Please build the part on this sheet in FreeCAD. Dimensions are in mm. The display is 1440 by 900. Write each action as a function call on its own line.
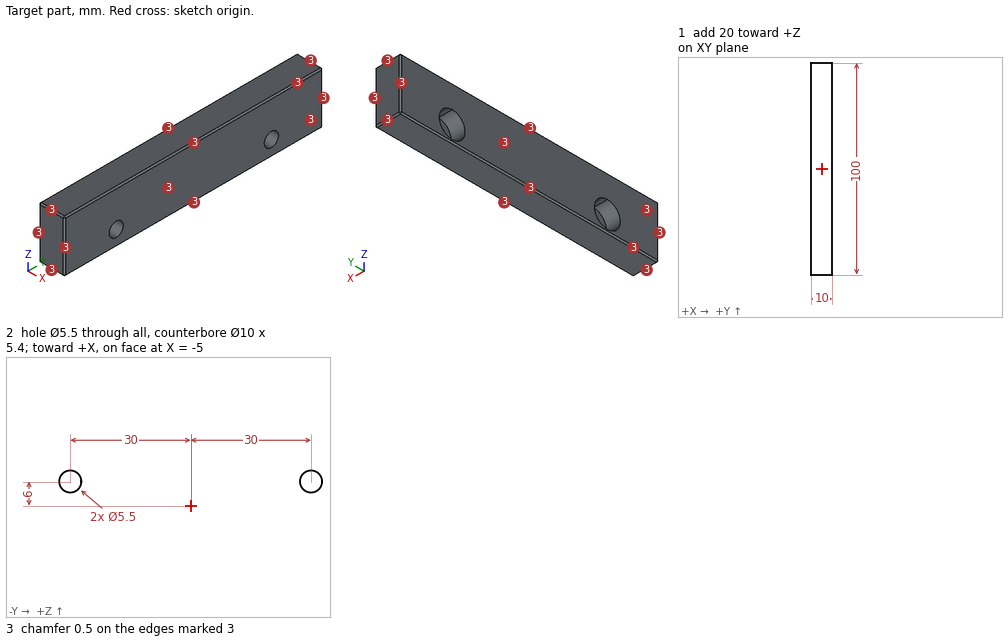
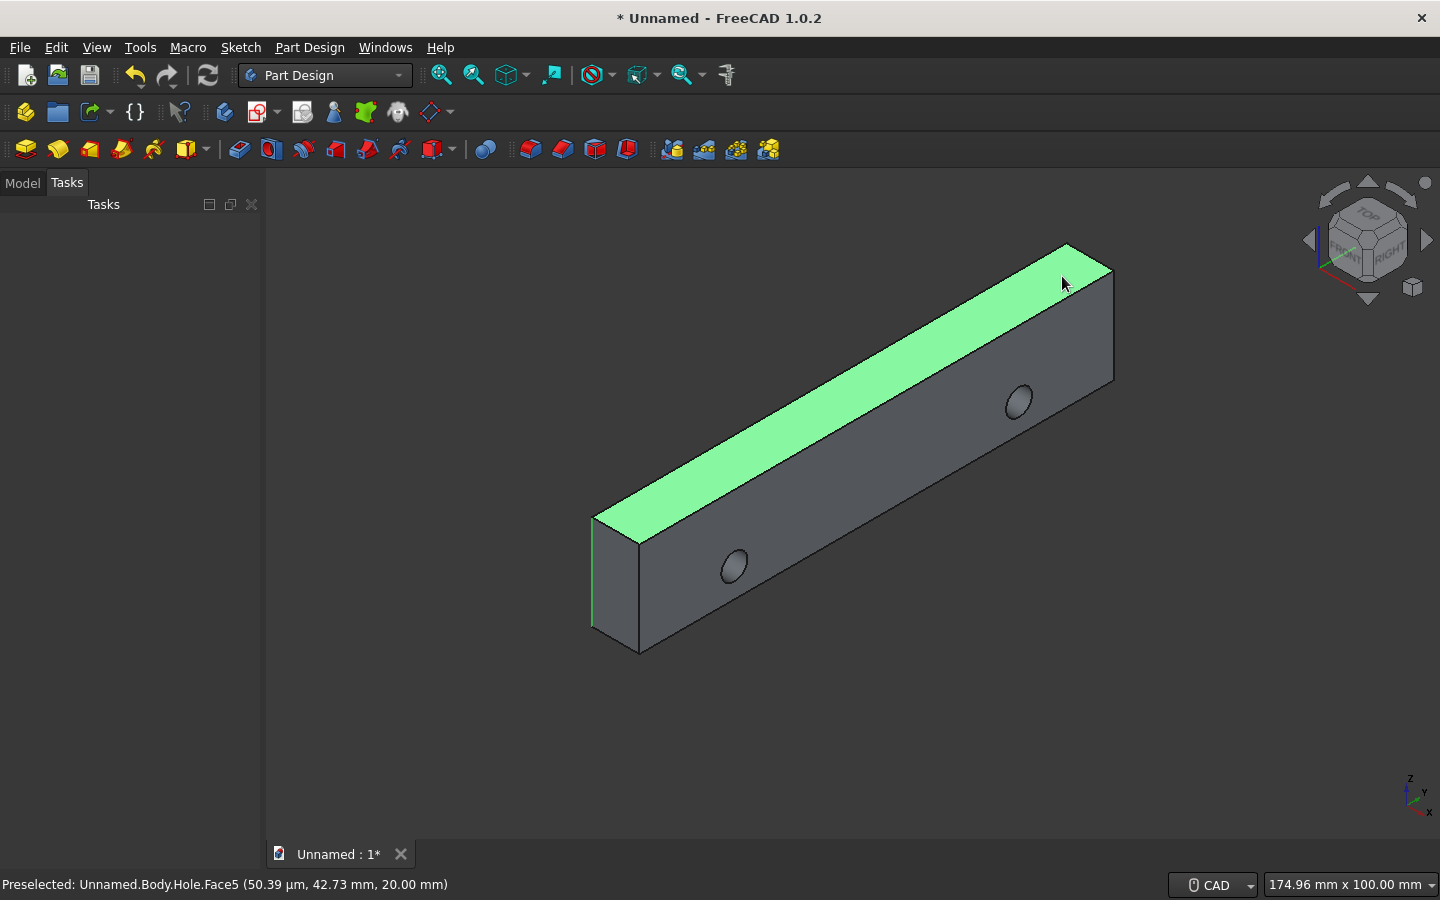
click(639, 598, ctrl)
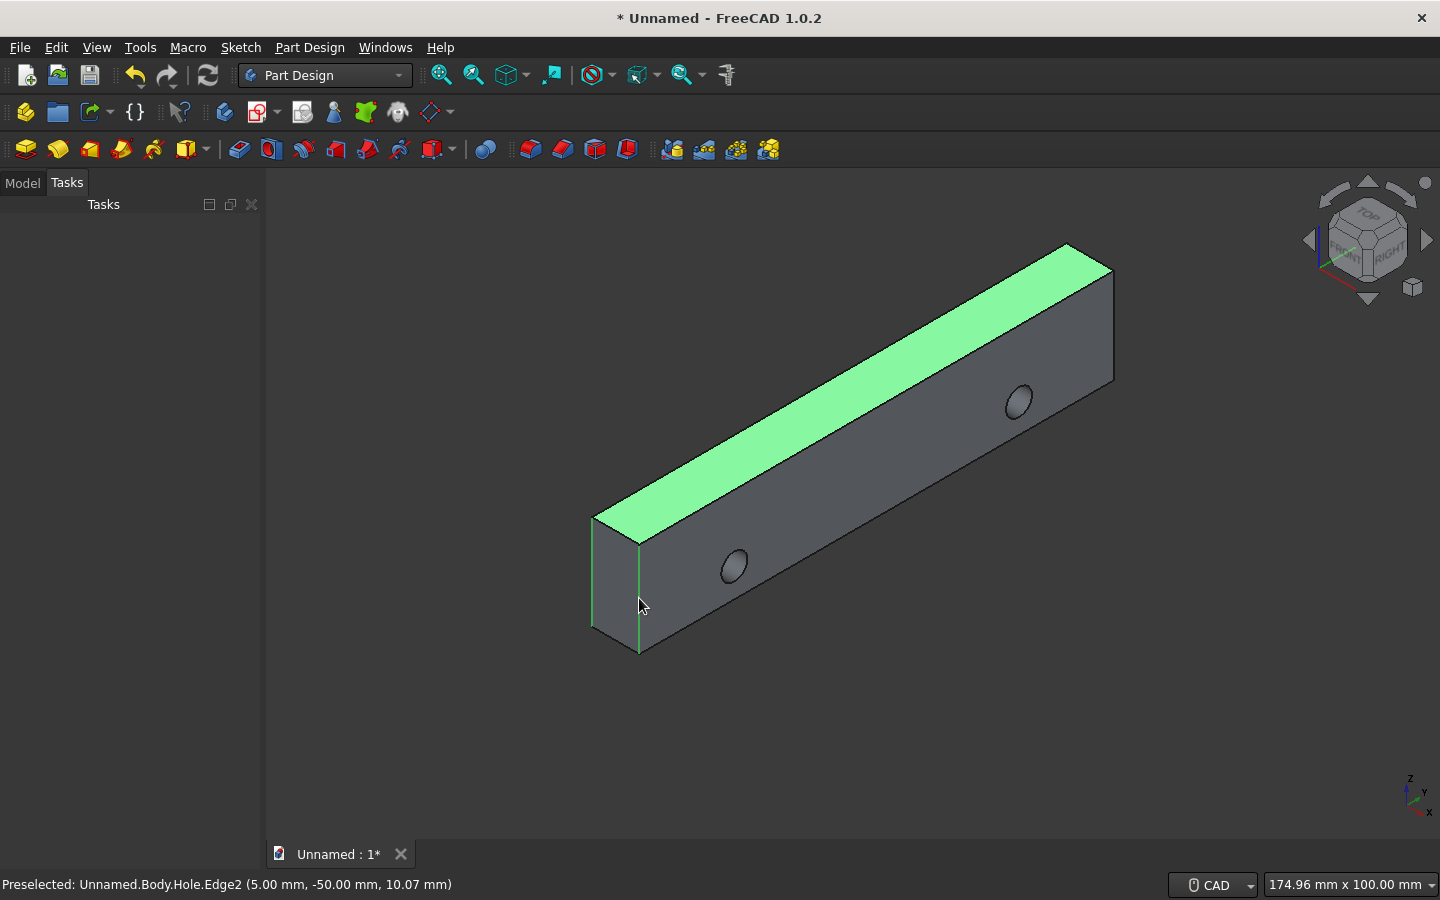
key(2)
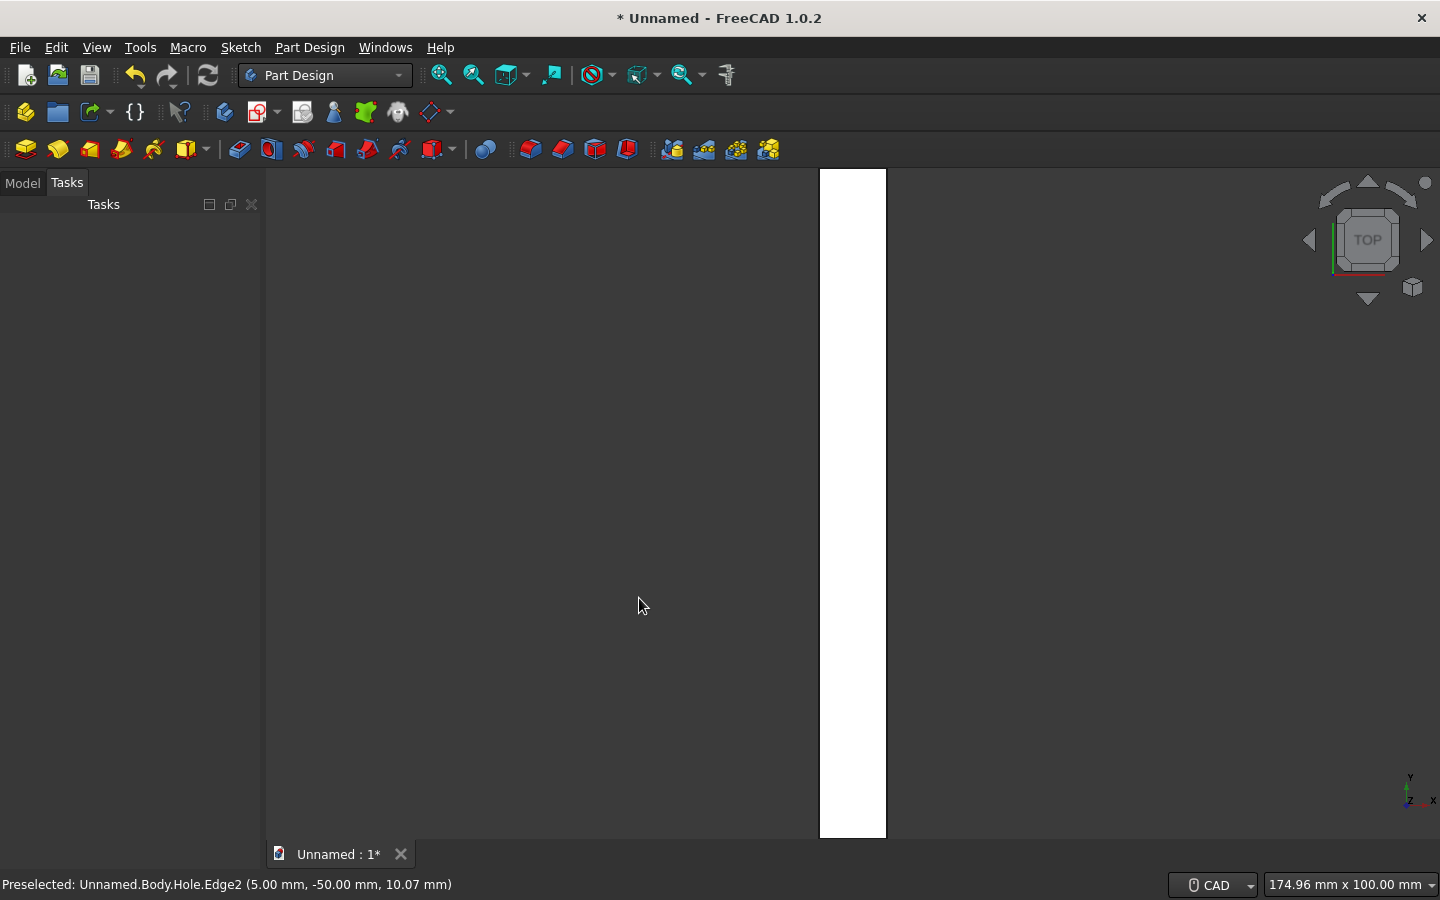
click(442, 76)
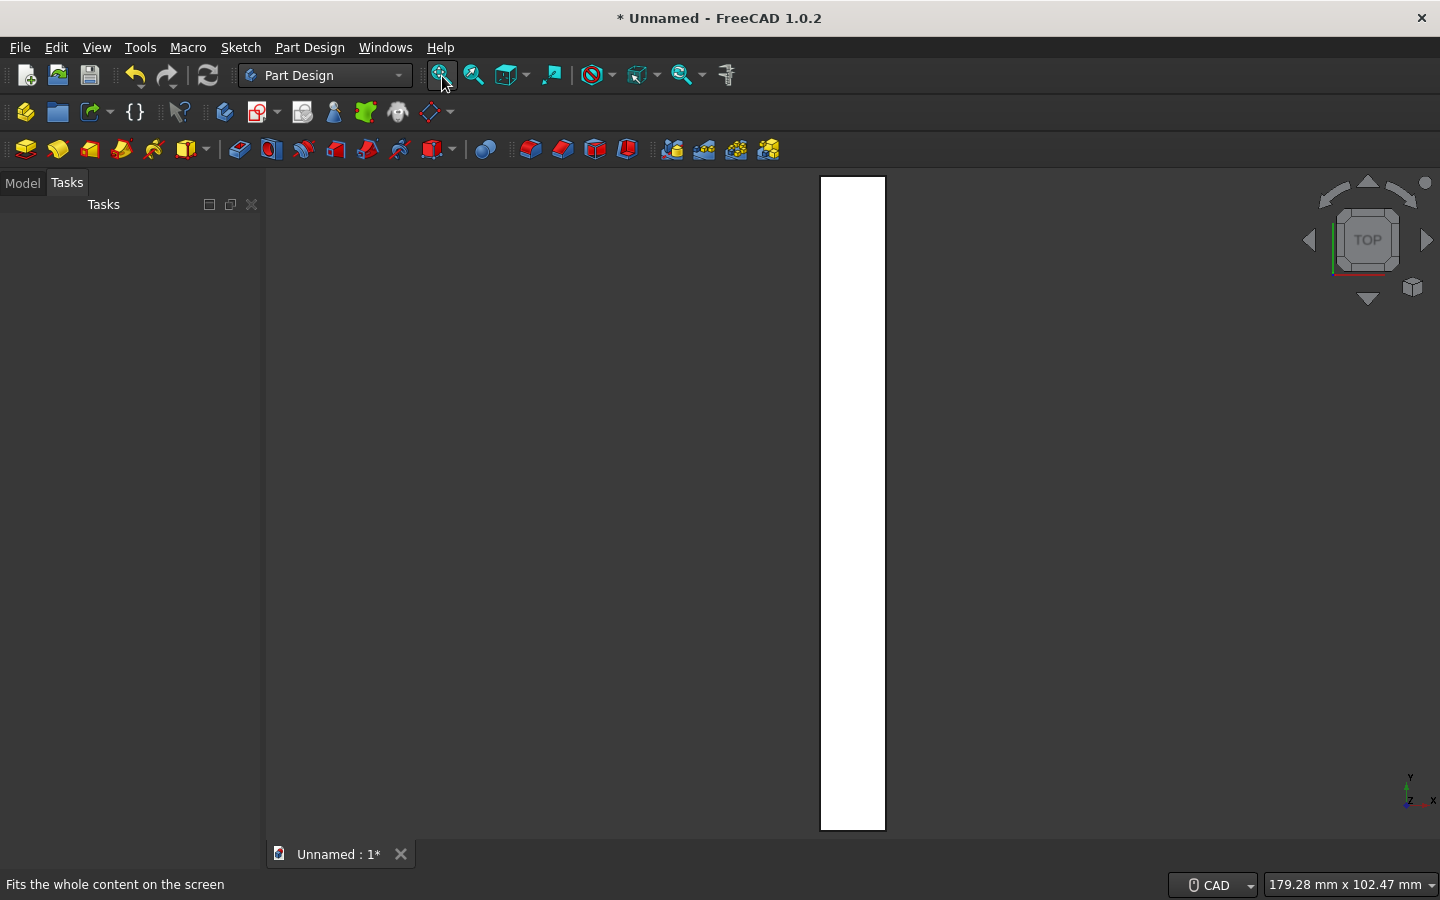
key(1)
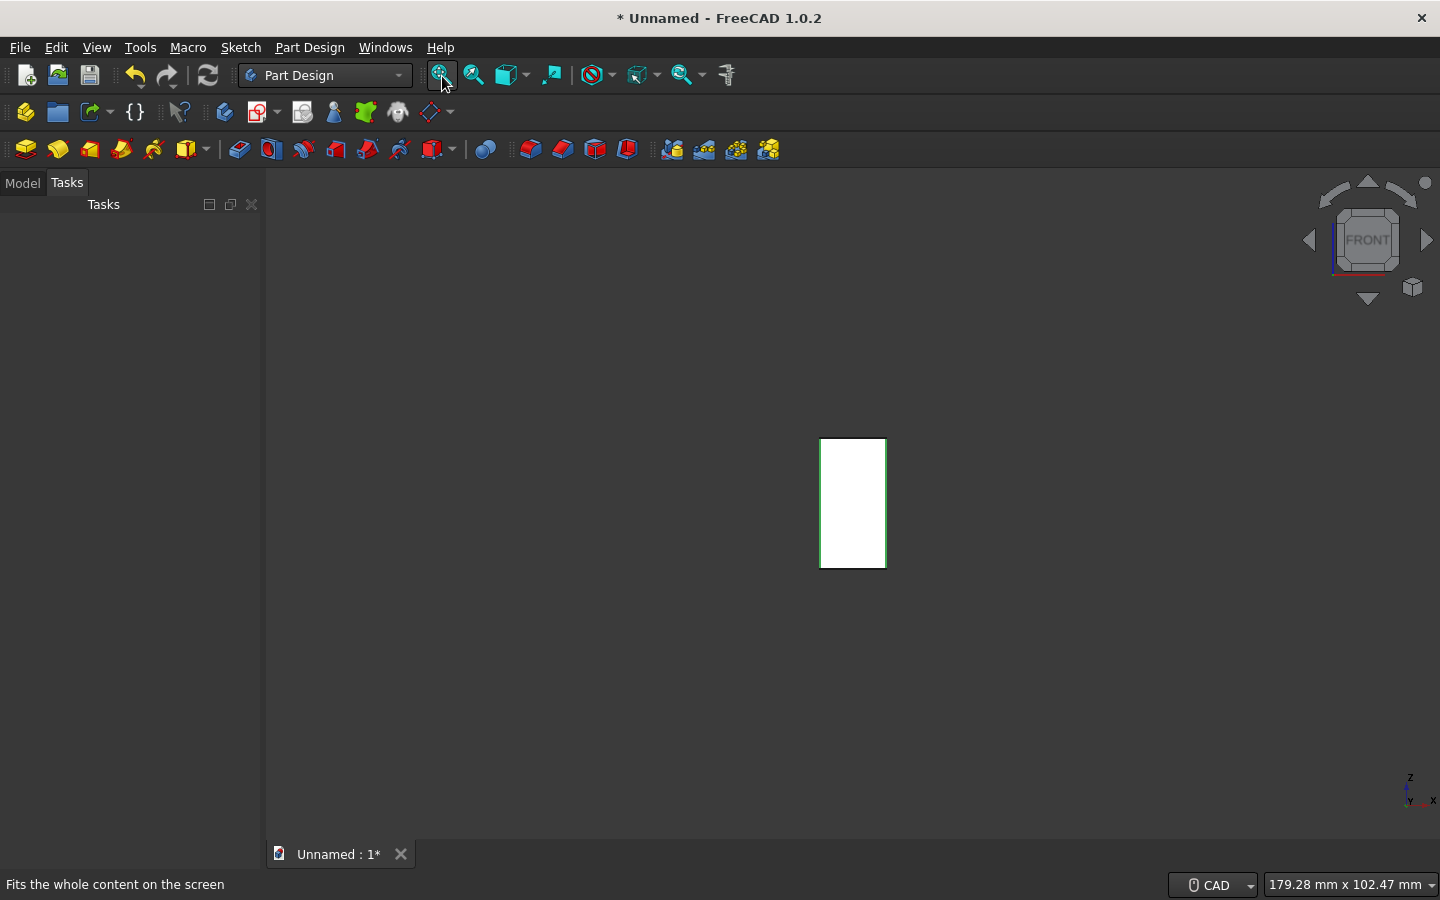
click(442, 76)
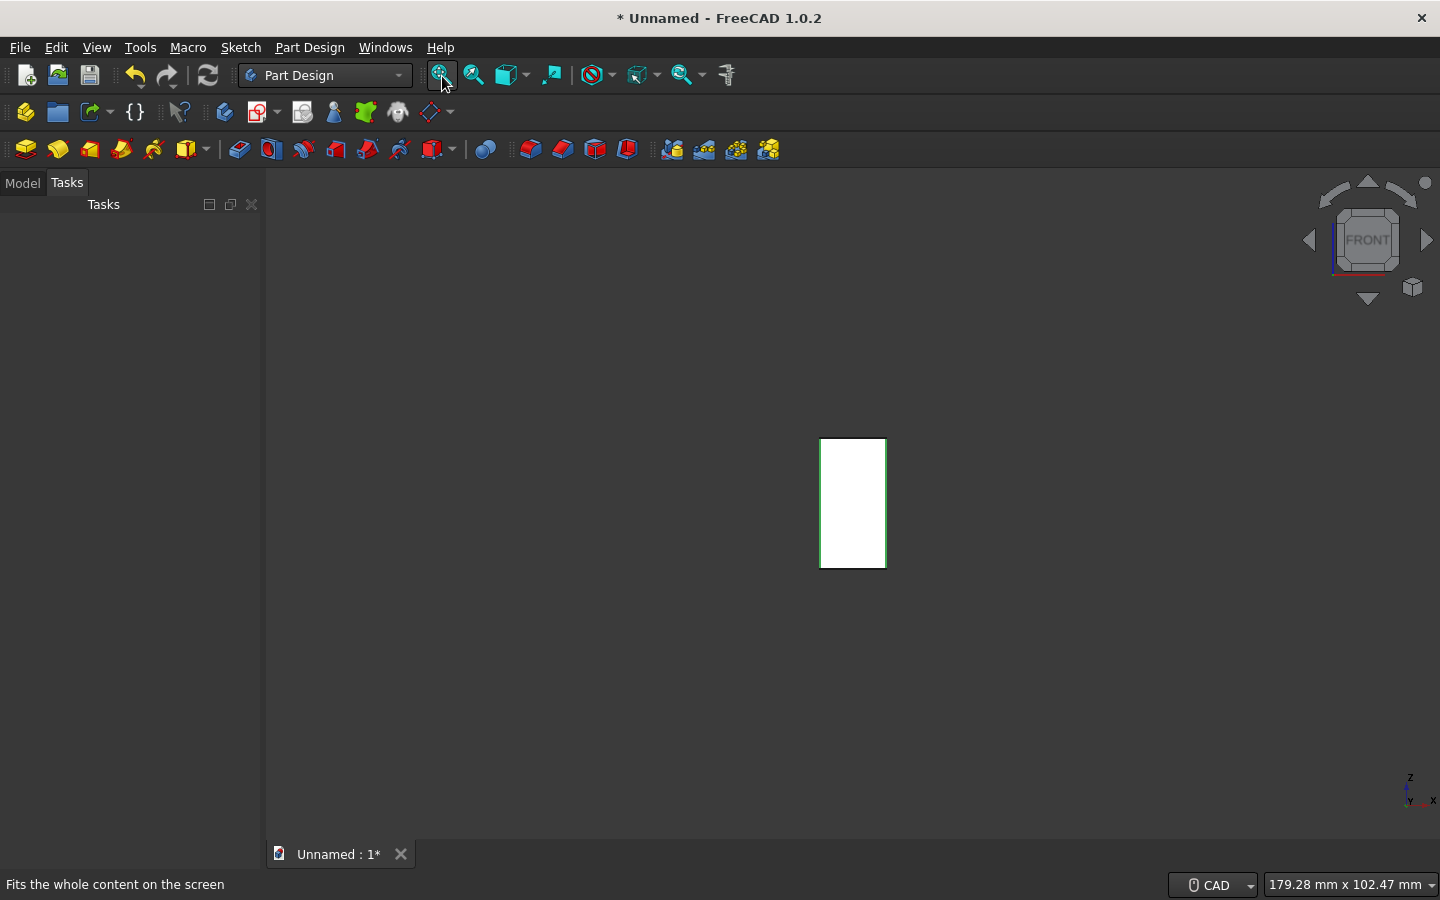
key(3)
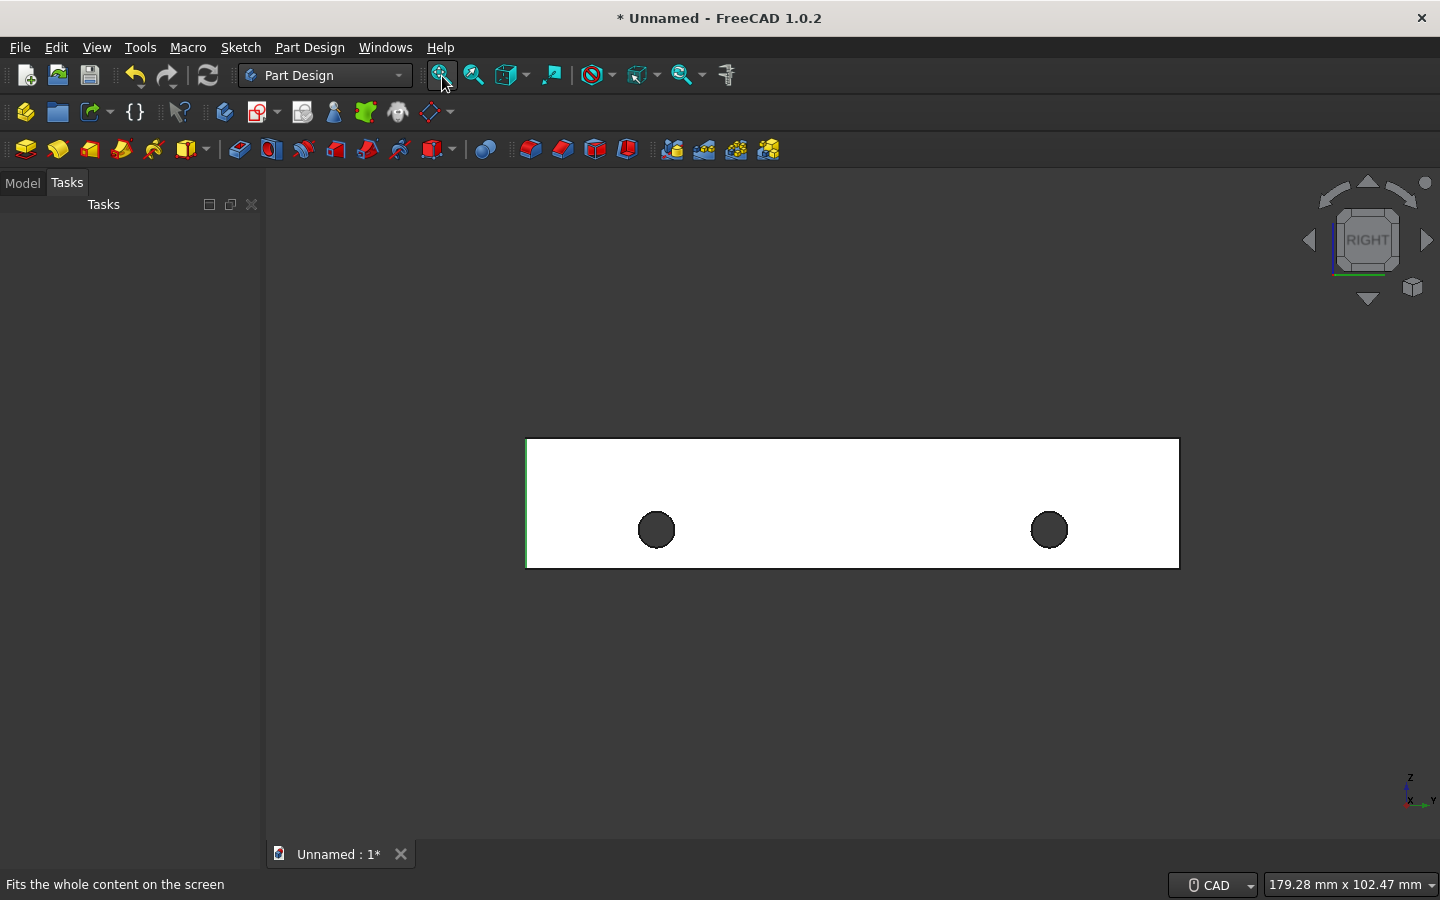
click(1180, 502, ctrl)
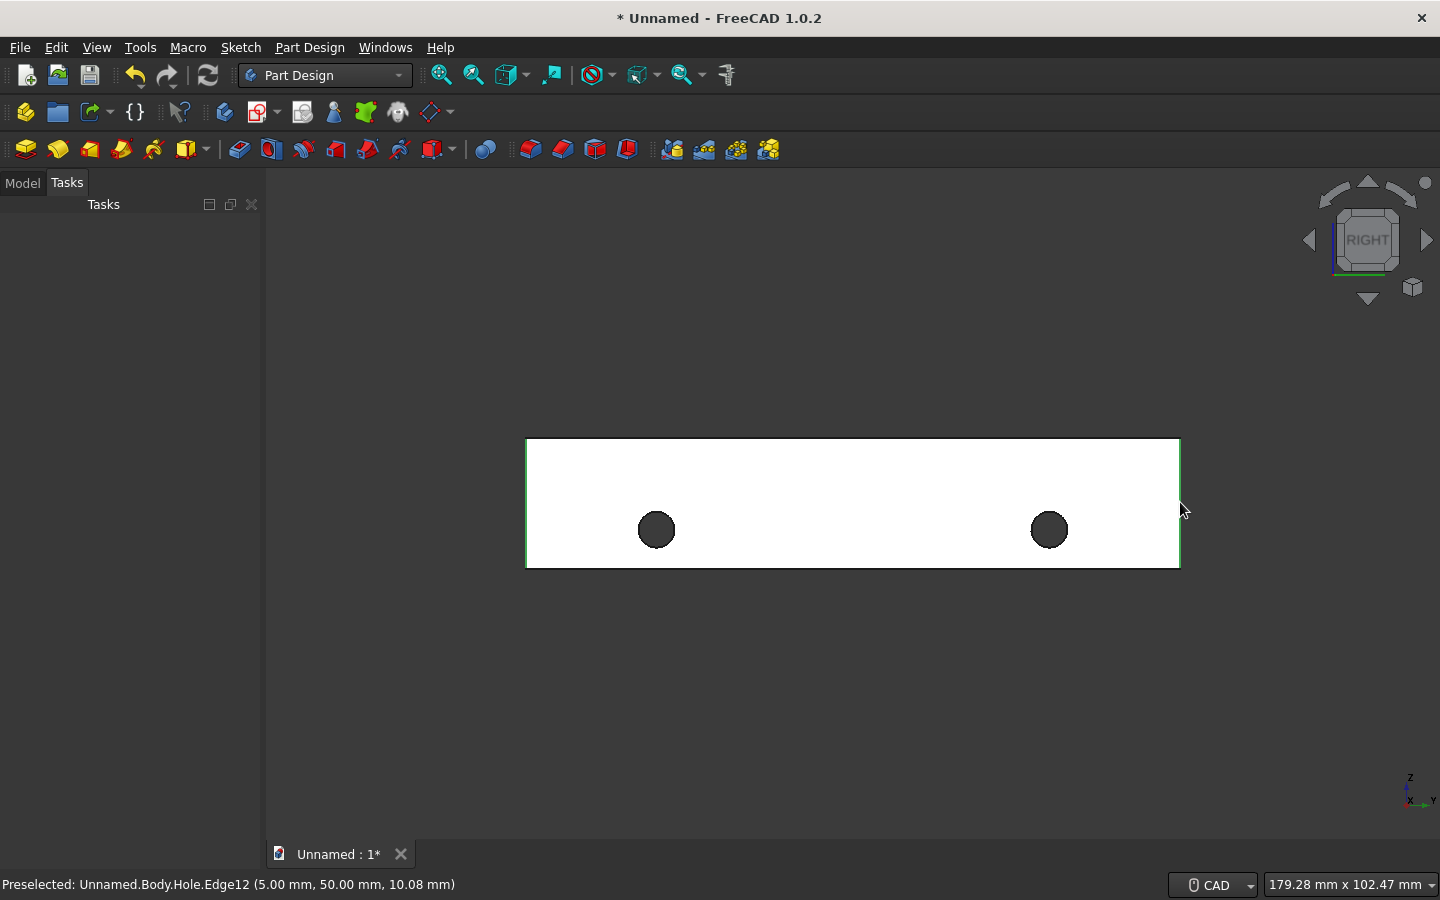
key(5)